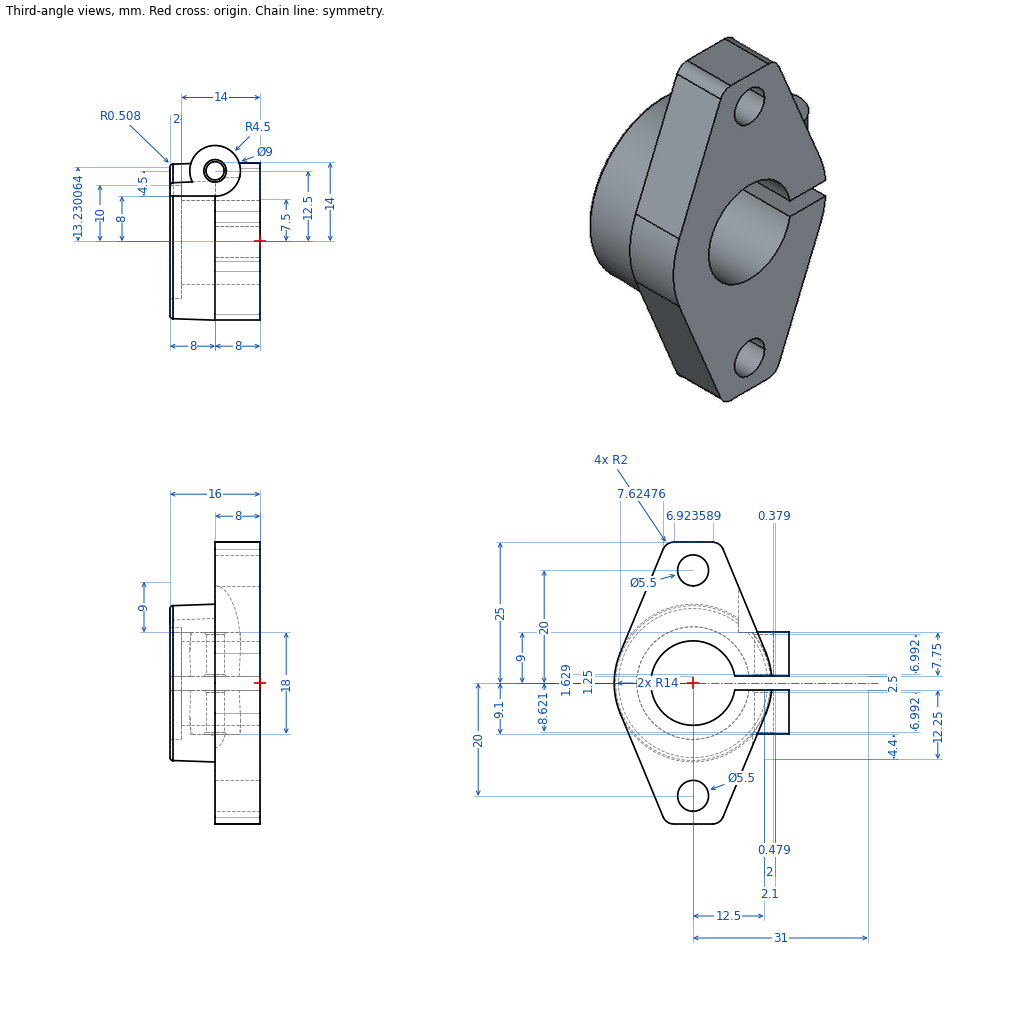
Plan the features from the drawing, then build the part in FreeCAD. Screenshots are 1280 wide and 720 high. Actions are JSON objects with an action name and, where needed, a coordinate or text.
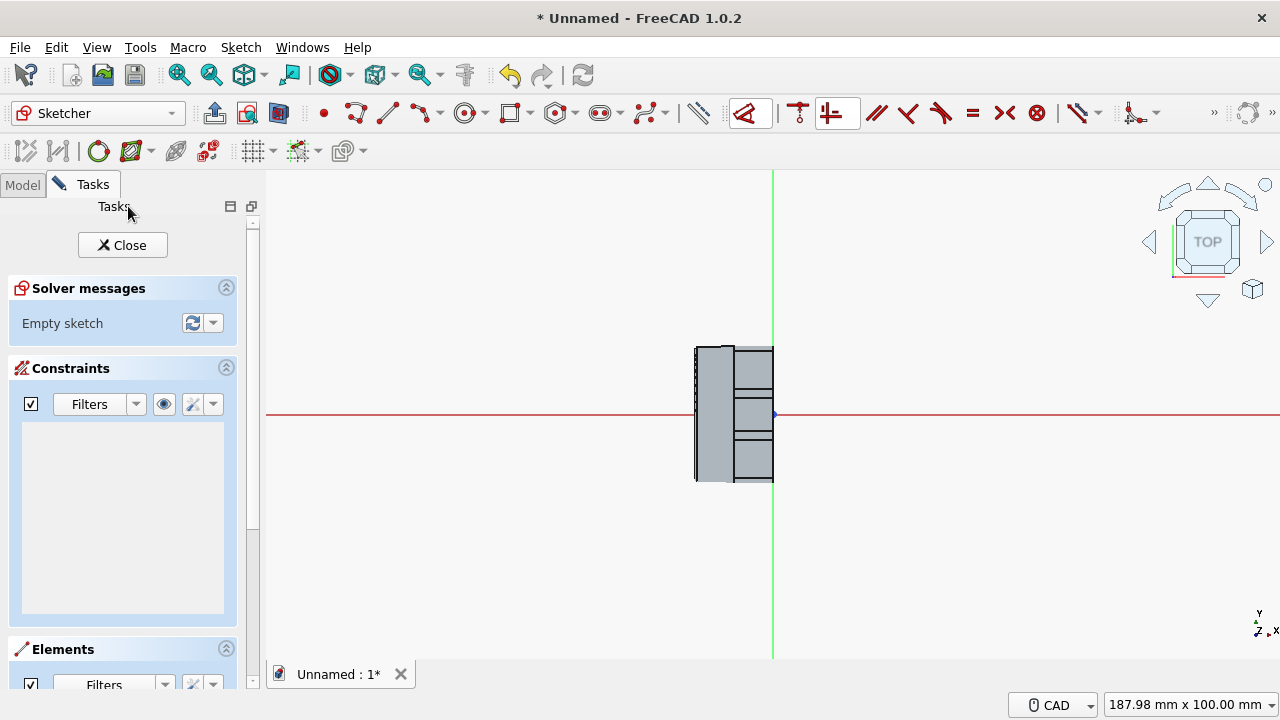
{"action": "left_click", "coordinate": [280, 114]}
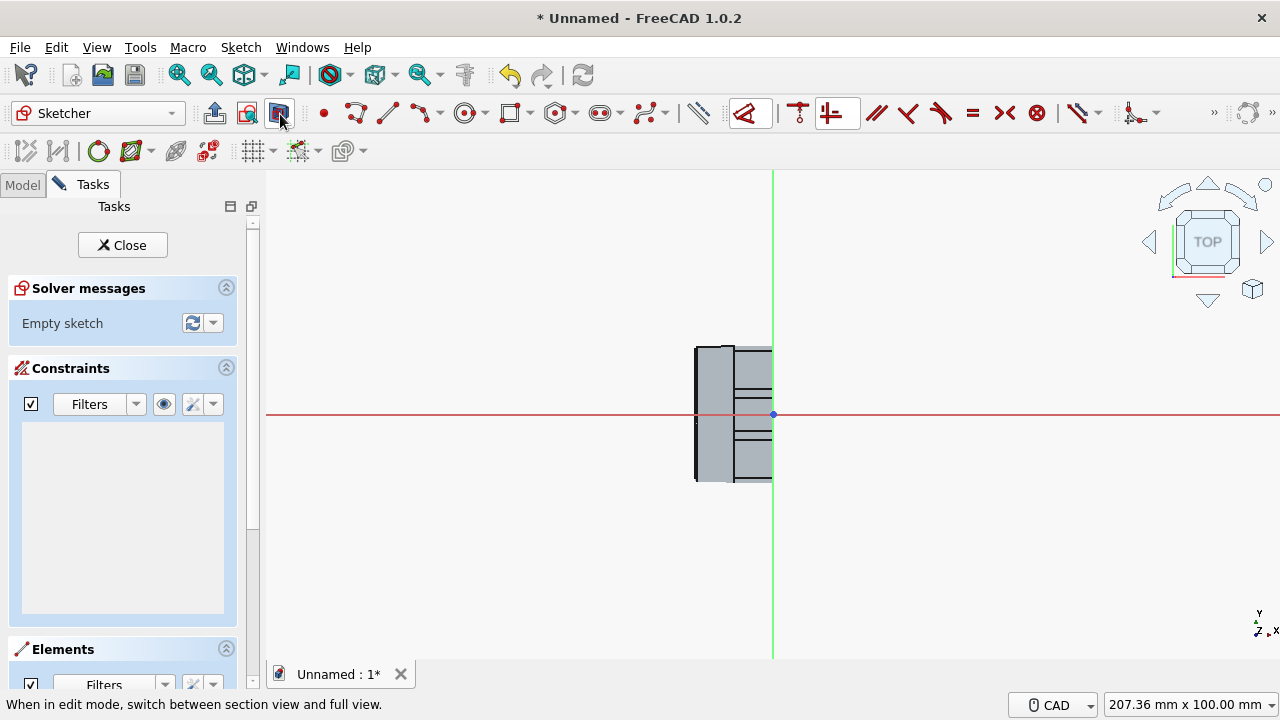
{"action": "scroll", "coordinate": [755, 359], "scroll_direction": "up", "scroll_amount": 7}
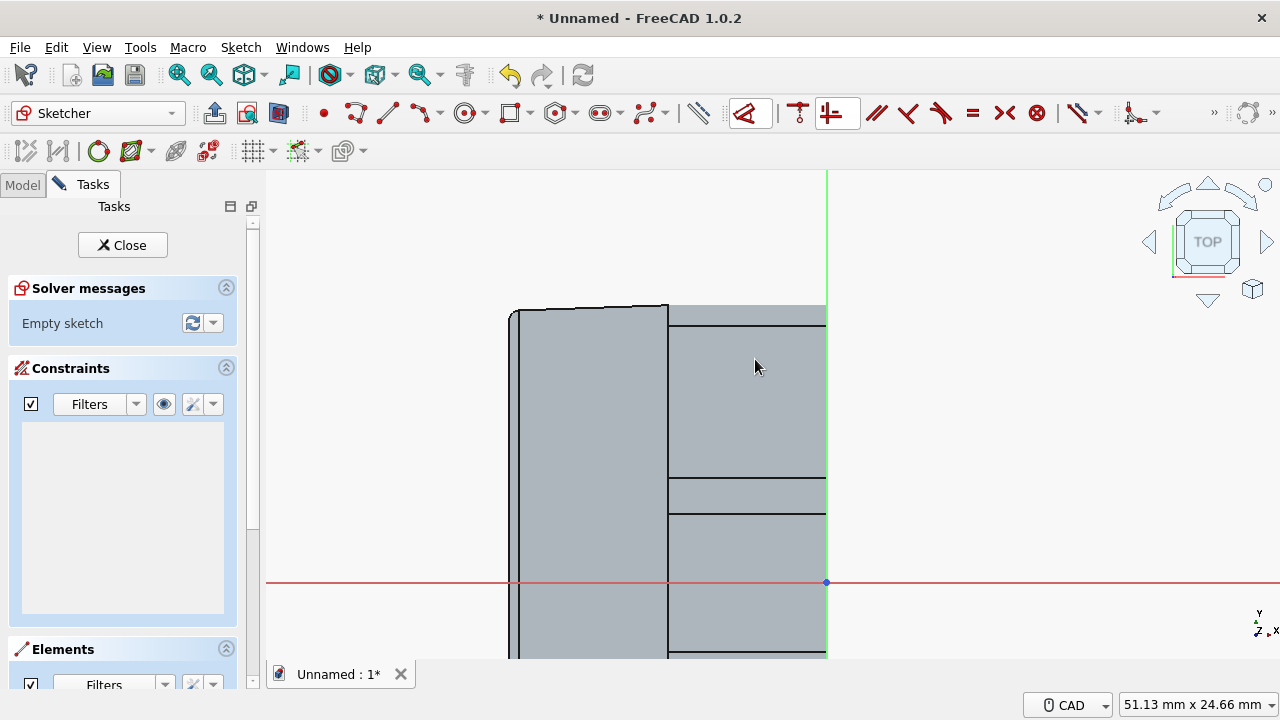
{"action": "left_click", "coordinate": [466, 114]}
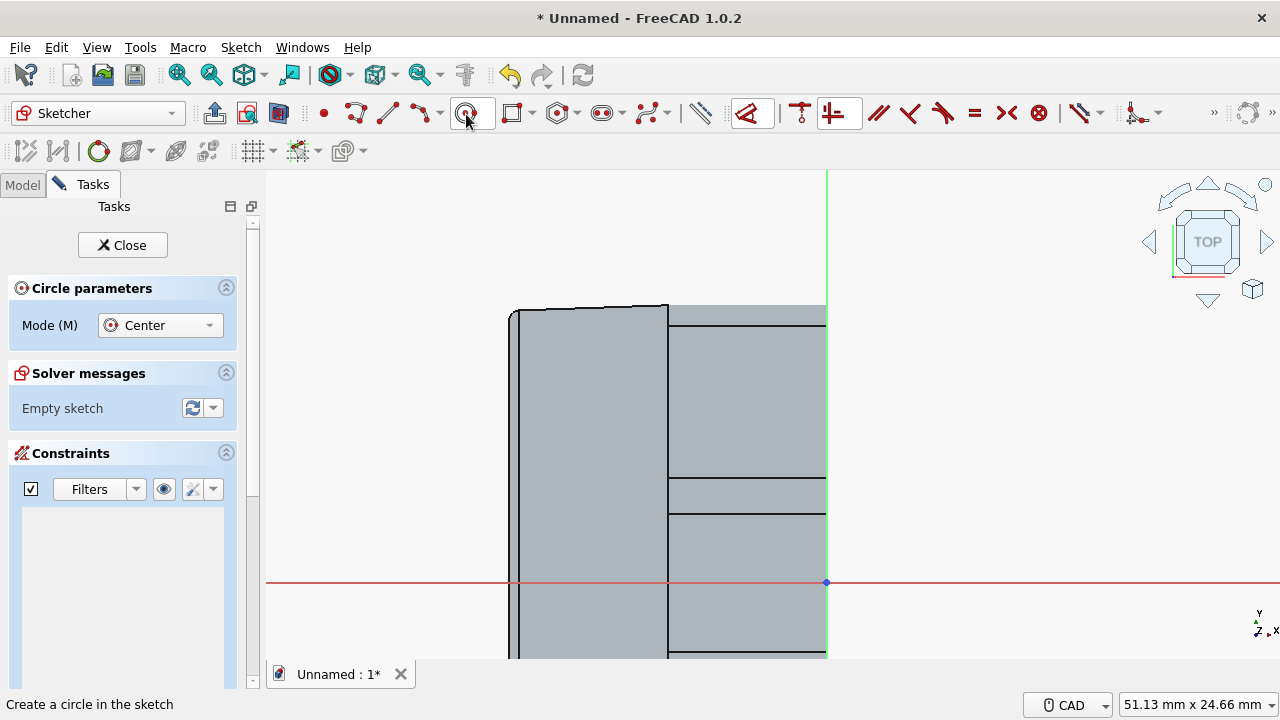
{"action": "left_click", "coordinate": [668, 335]}
{"action": "mouse_move", "coordinate": [731, 272]}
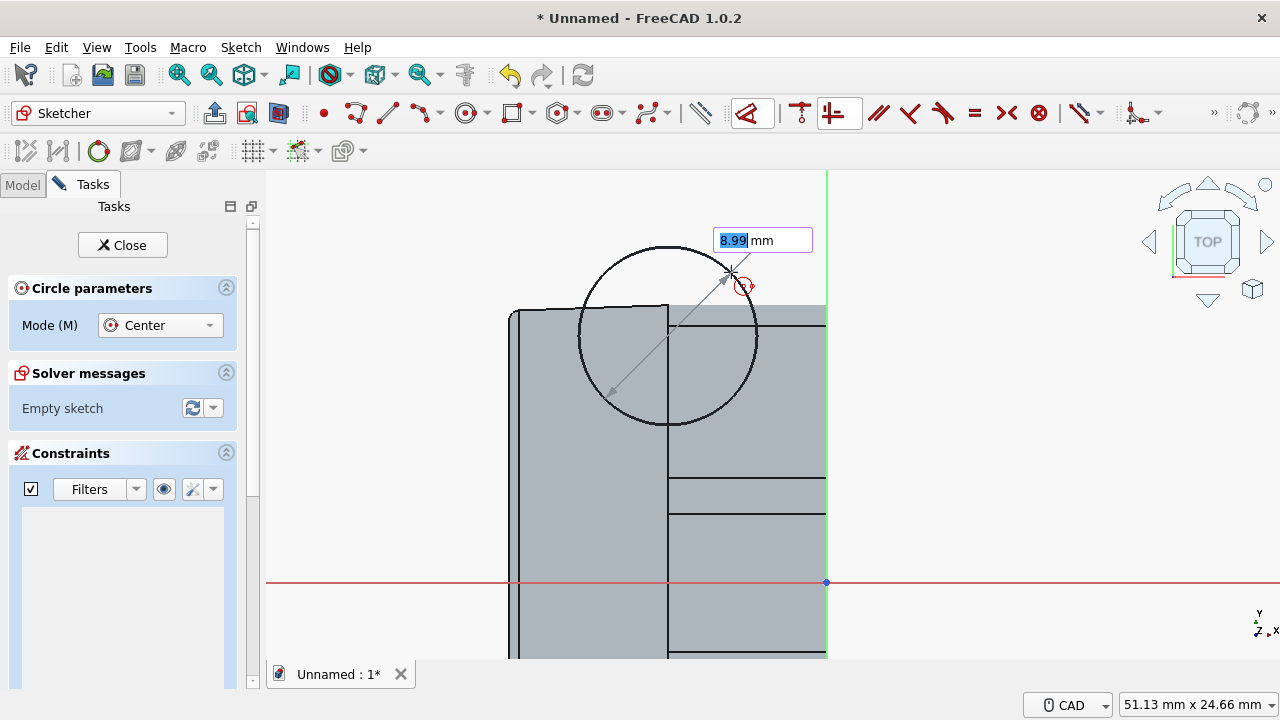
{"action": "type", "text": "9"}
{"action": "key", "text": "Return"}
{"action": "key", "text": "Escape"}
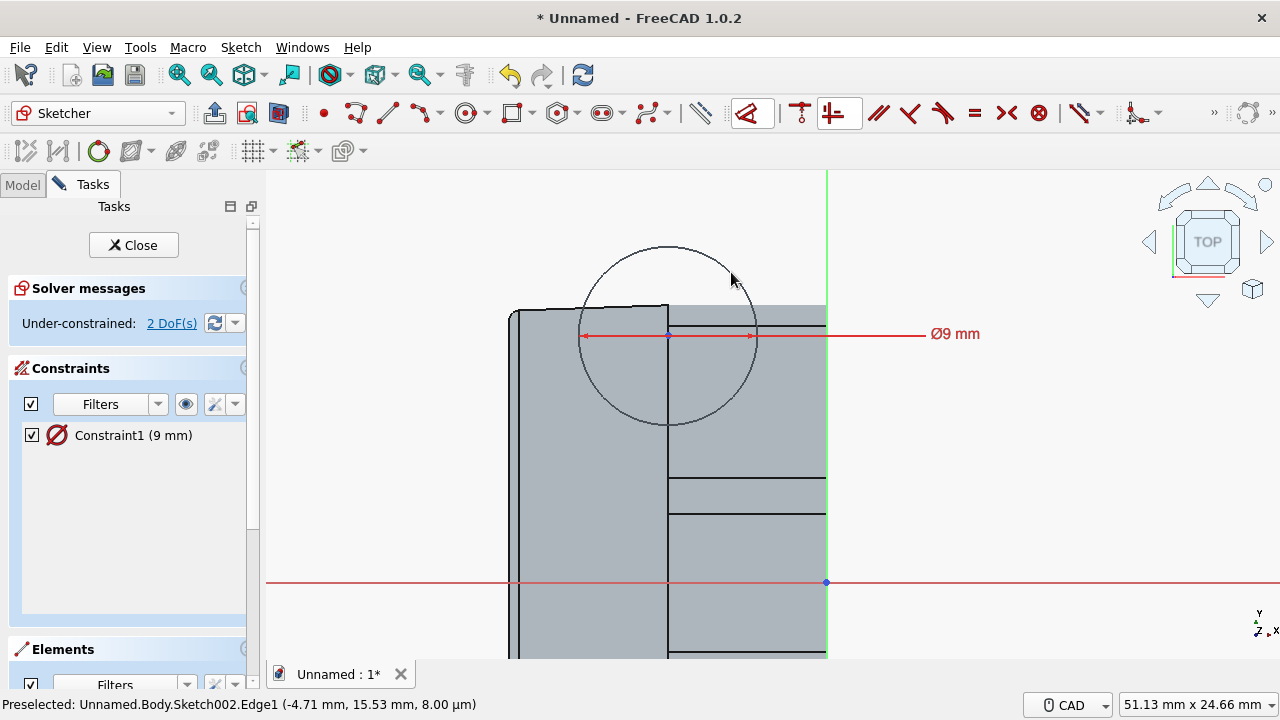
{"action": "left_click", "coordinate": [668, 336]}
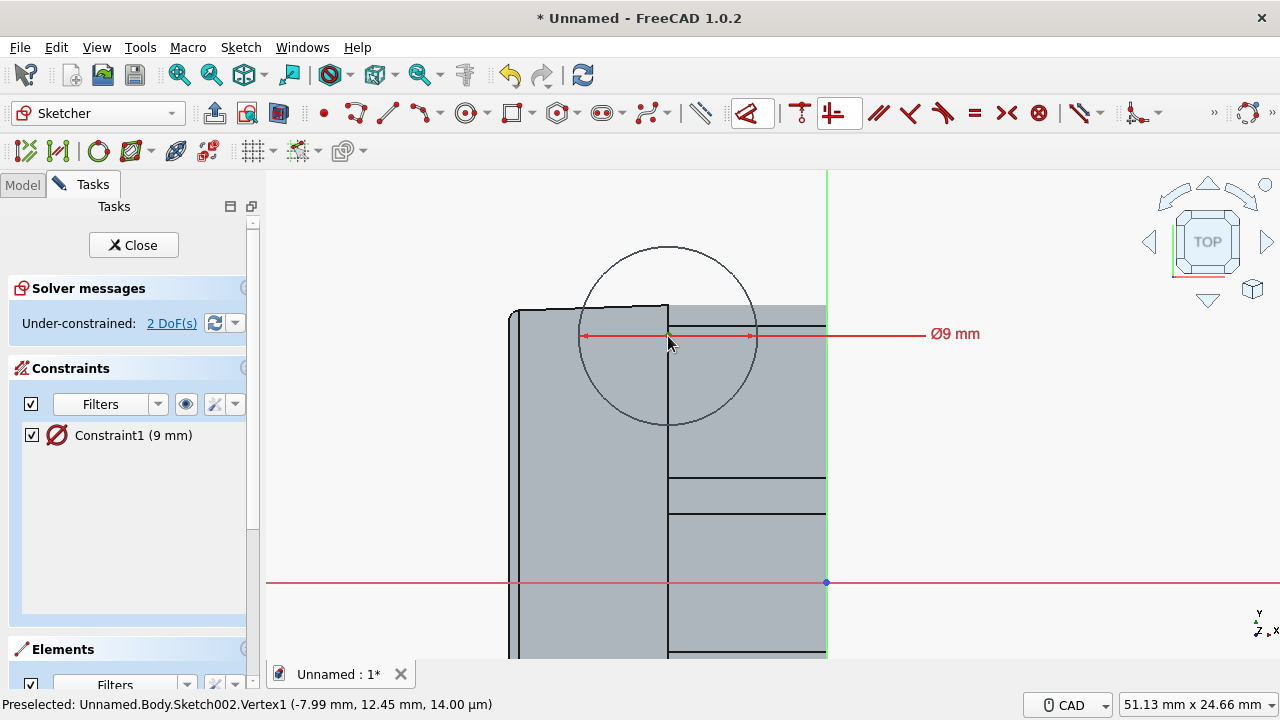
{"action": "key", "text": "l"}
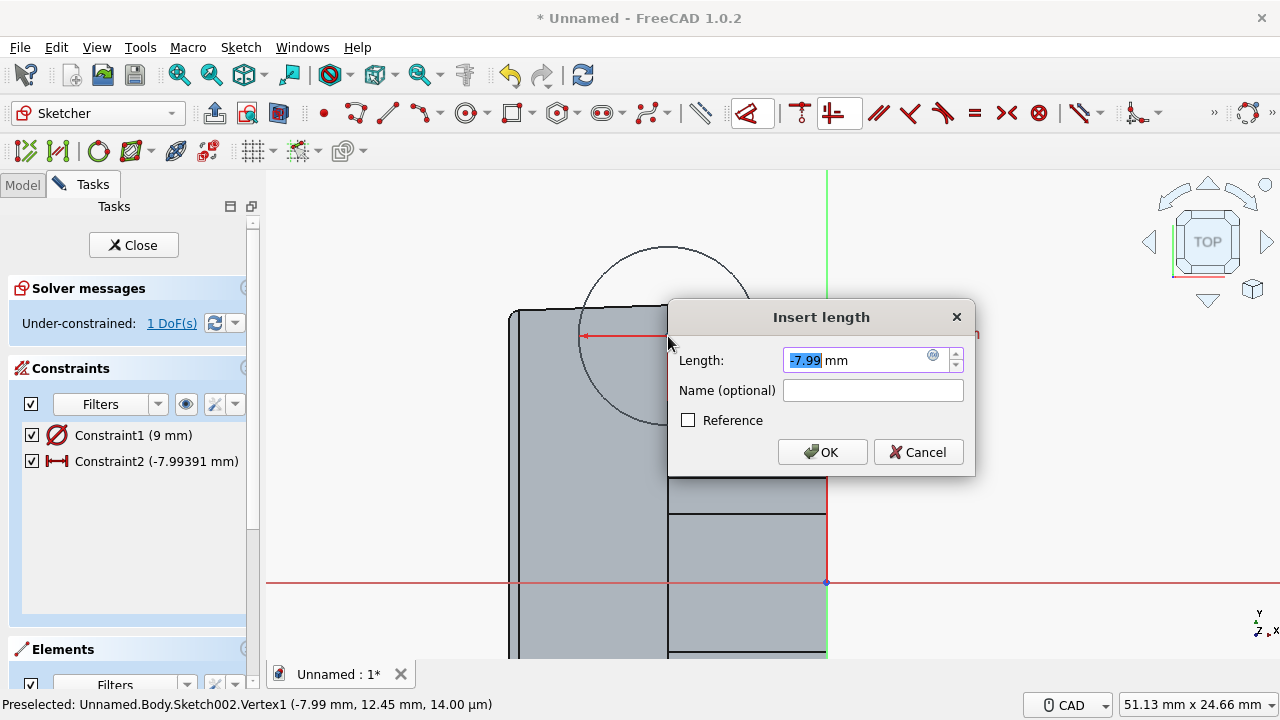
{"action": "type", "text": "-8"}
{"action": "key", "text": "Return"}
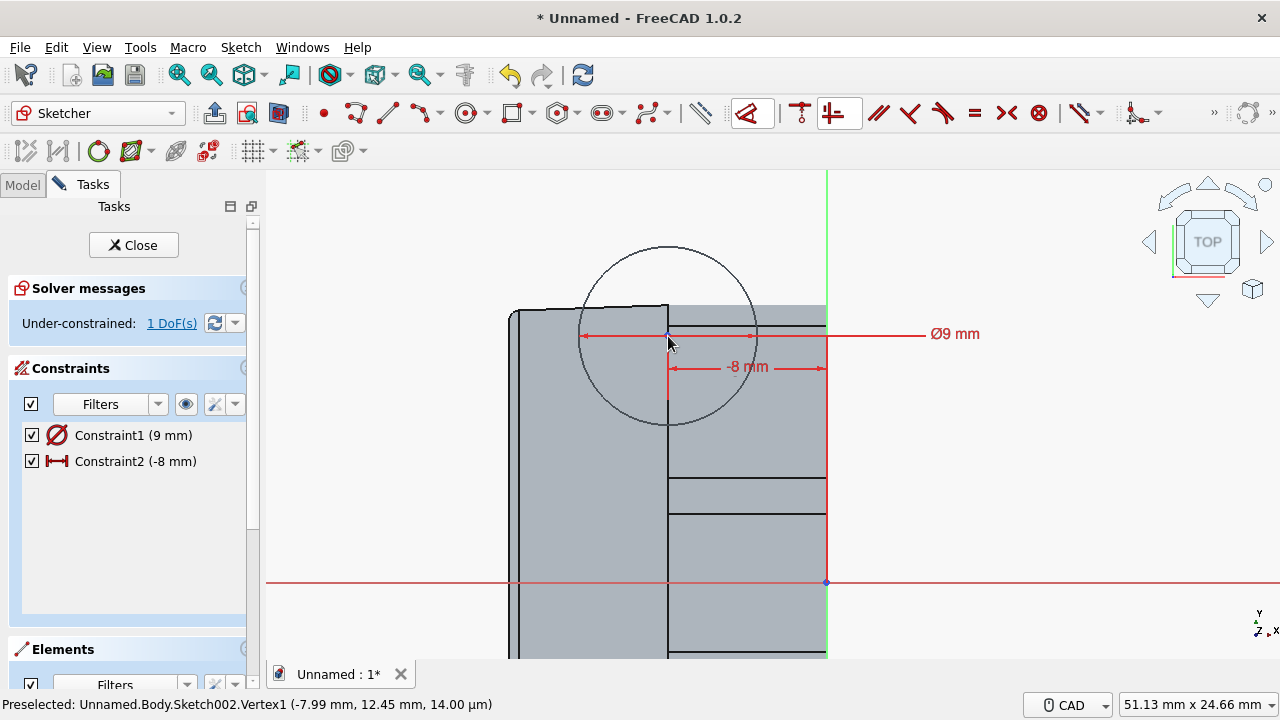
{"action": "left_click", "coordinate": [668, 336]}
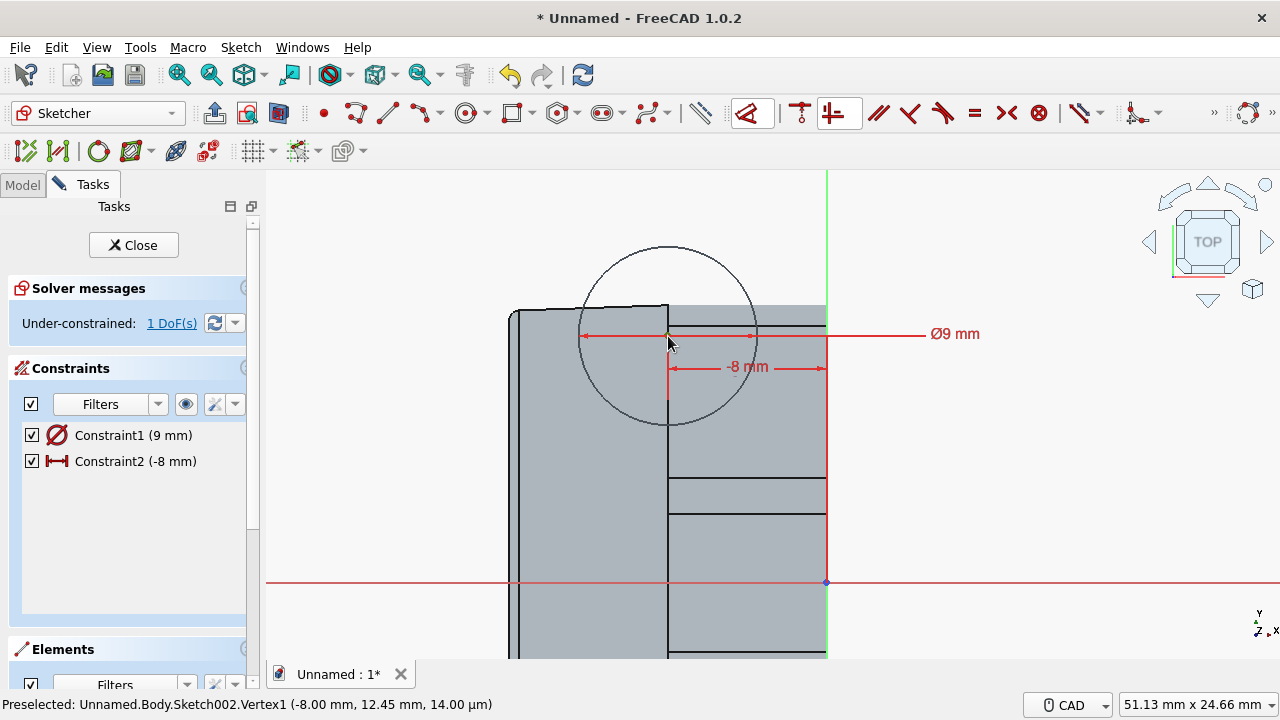
{"action": "left_click", "coordinate": [768, 114]}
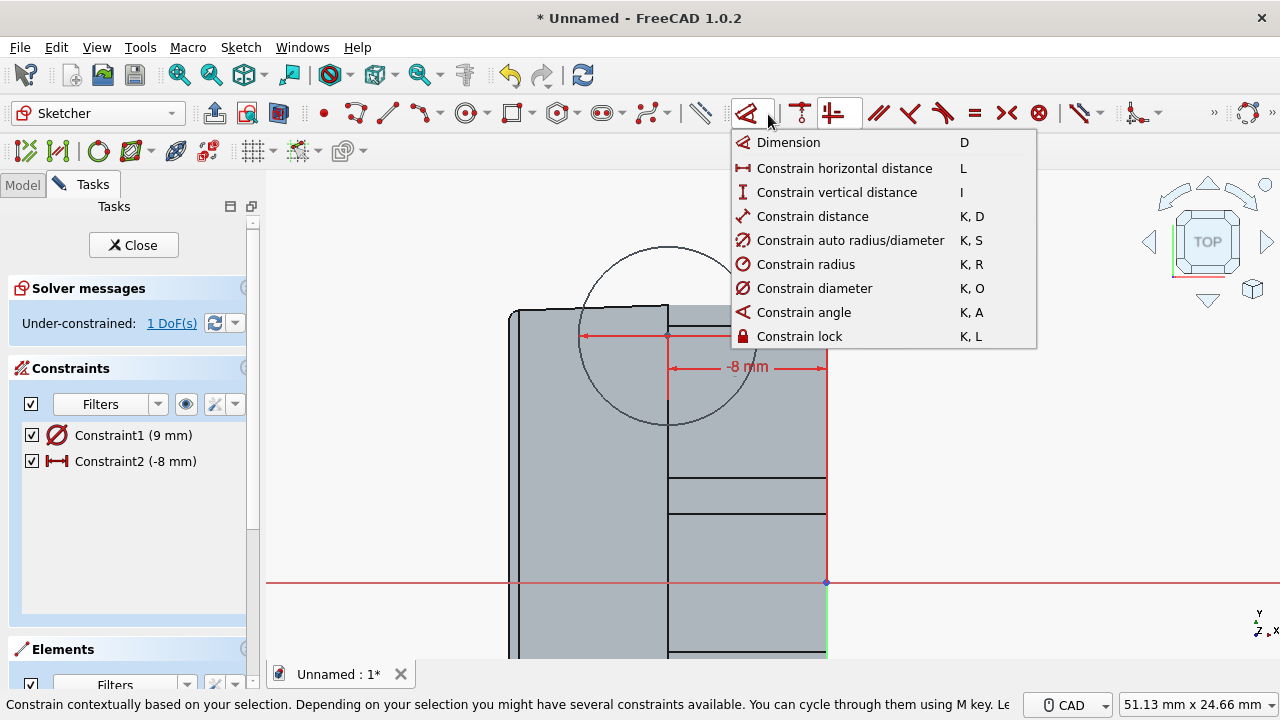
{"action": "left_click", "coordinate": [884, 192]}